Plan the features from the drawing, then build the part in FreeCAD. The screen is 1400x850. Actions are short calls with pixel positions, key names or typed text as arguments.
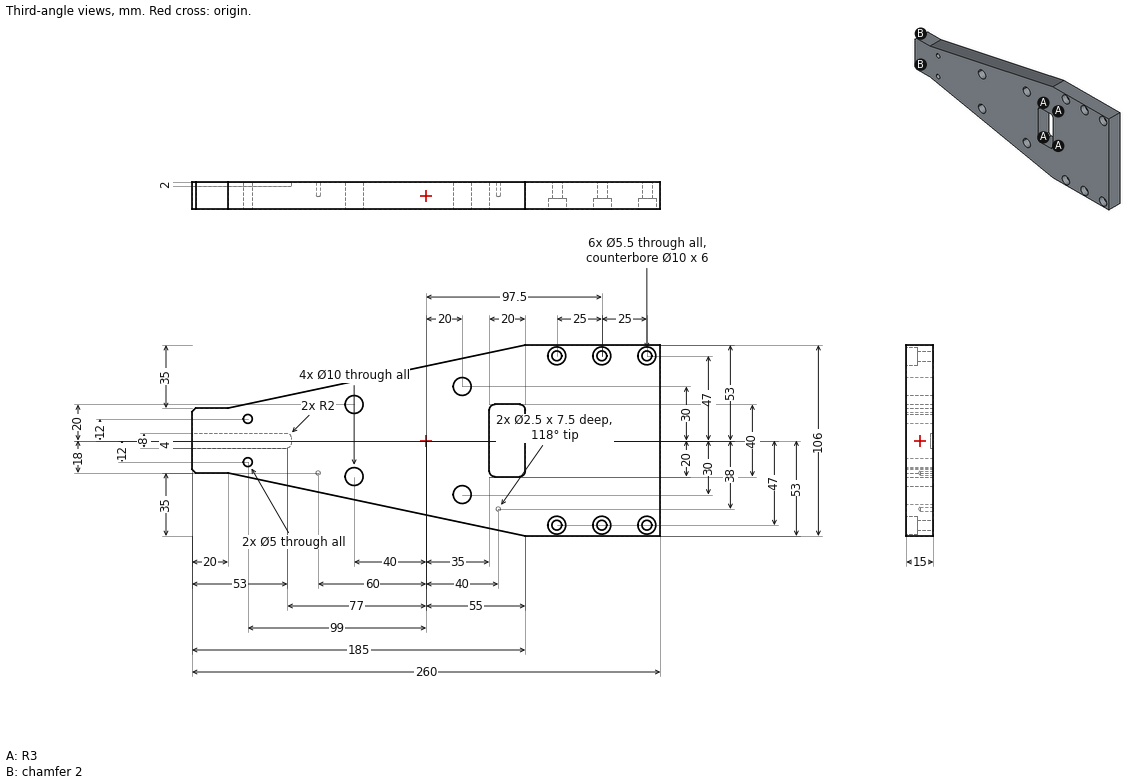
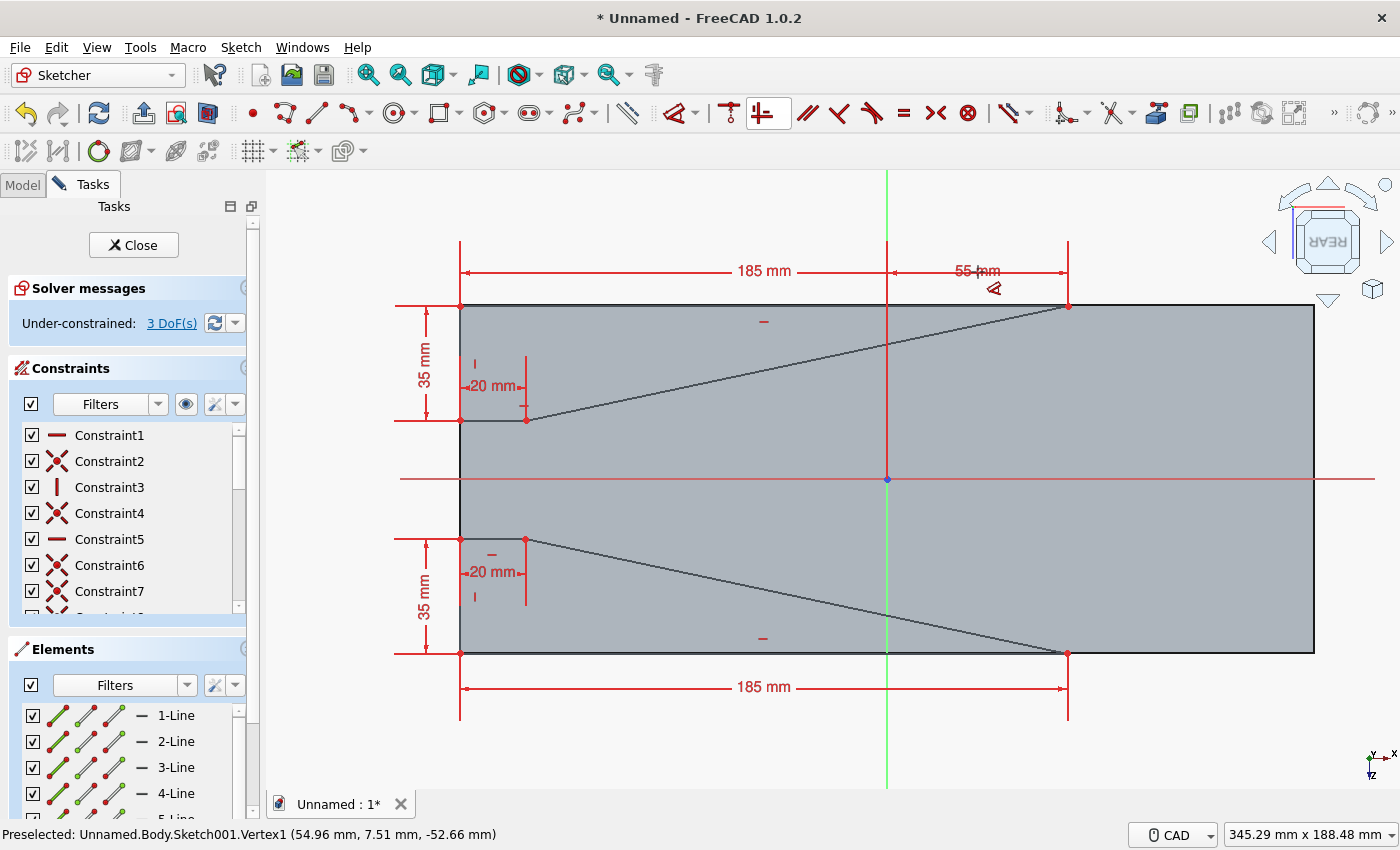
click(1068, 306)
click(1102, 393)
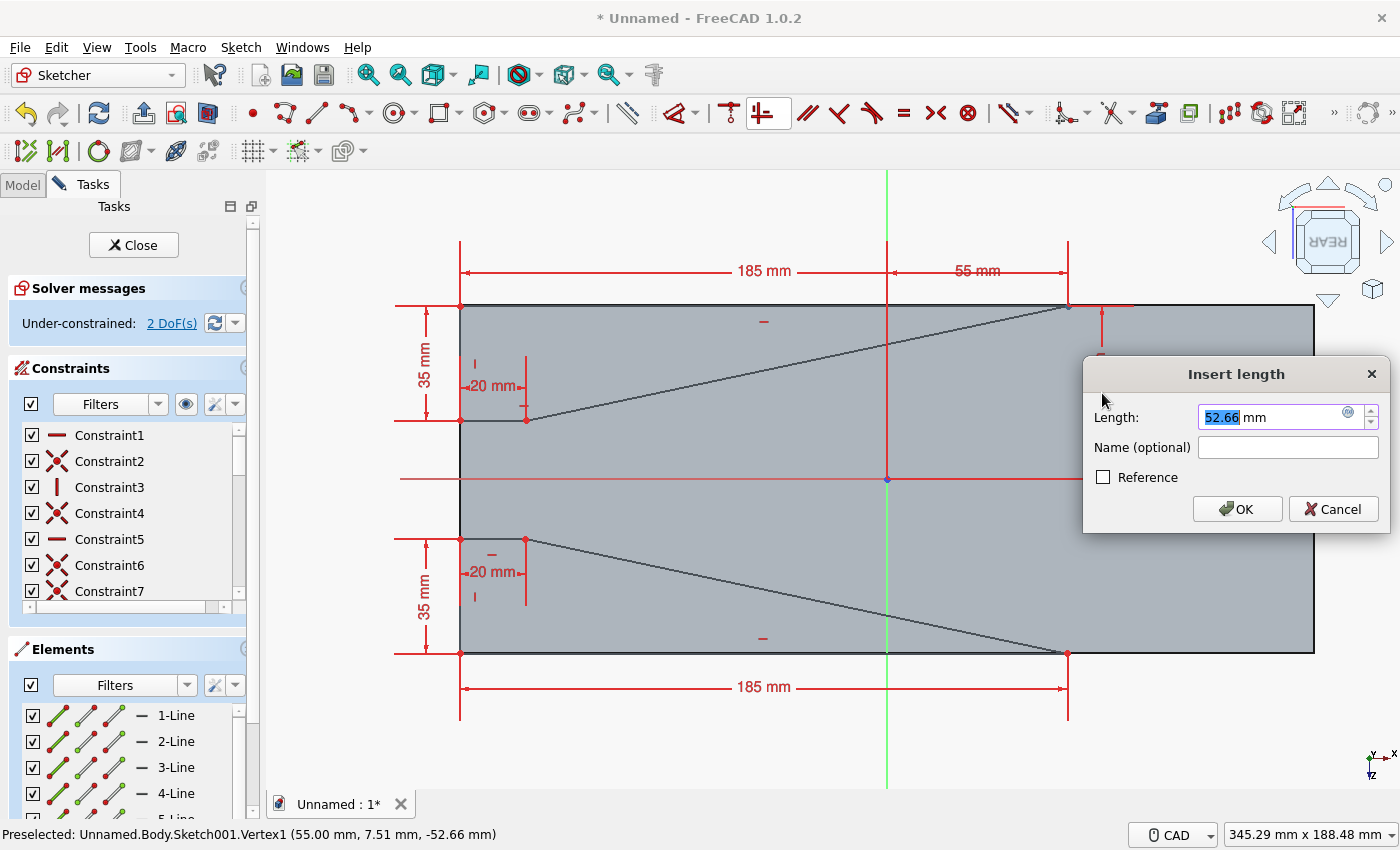
text(53)
key(Return)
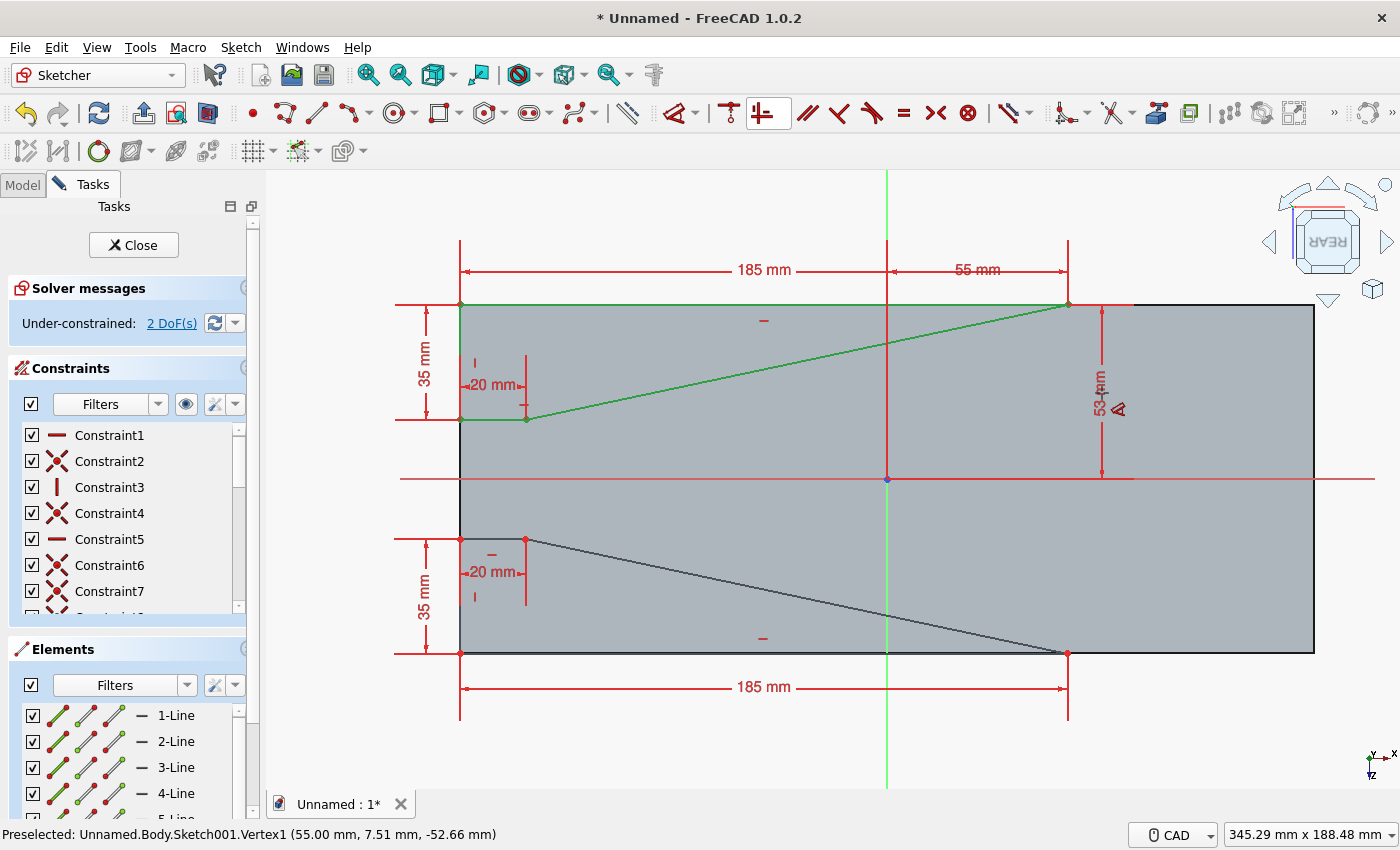
click(1068, 654)
click(978, 688)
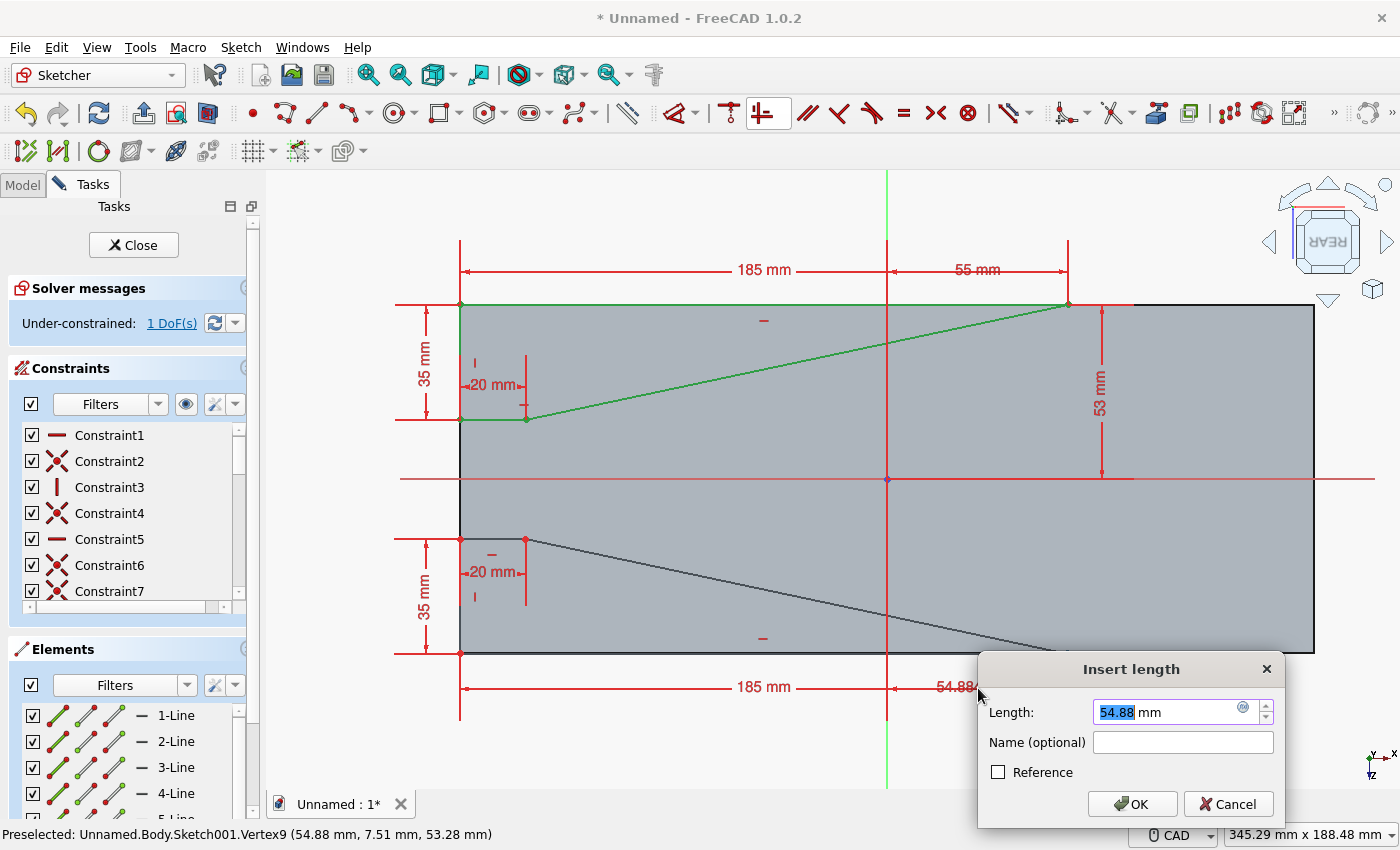
text(55)
key(Return)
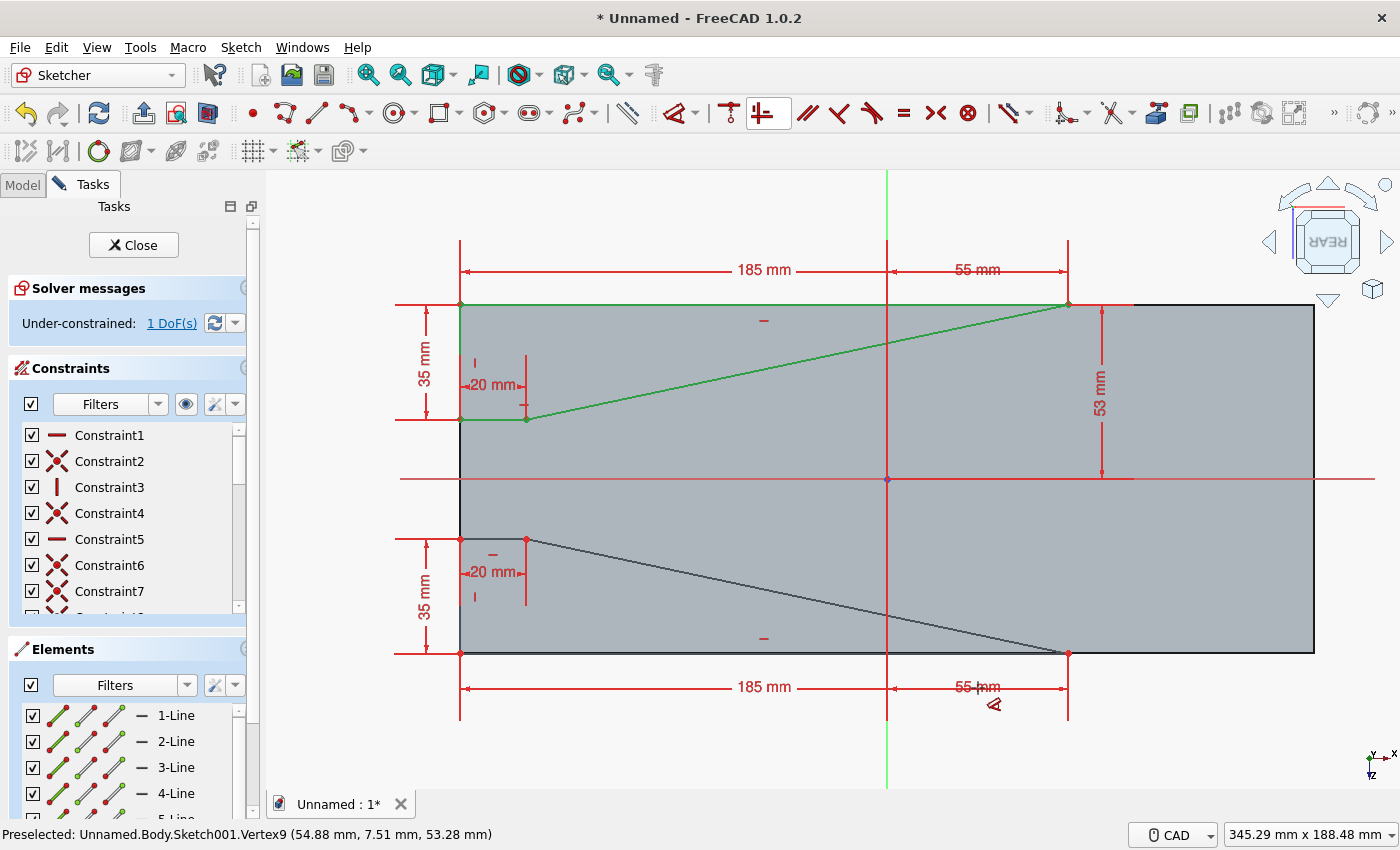
click(1068, 654)
click(1102, 567)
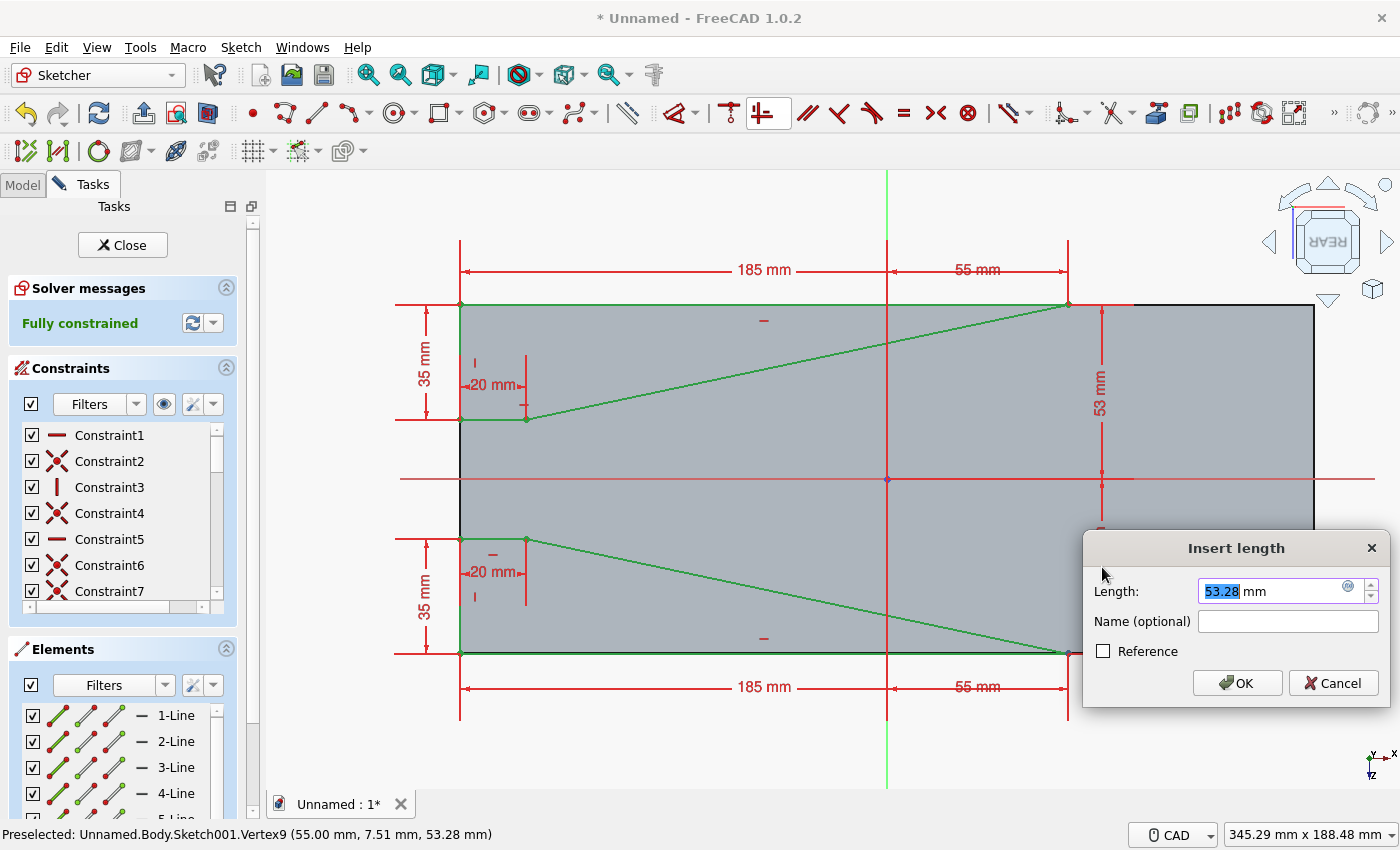
text(53)
key(Return)
key(Escape)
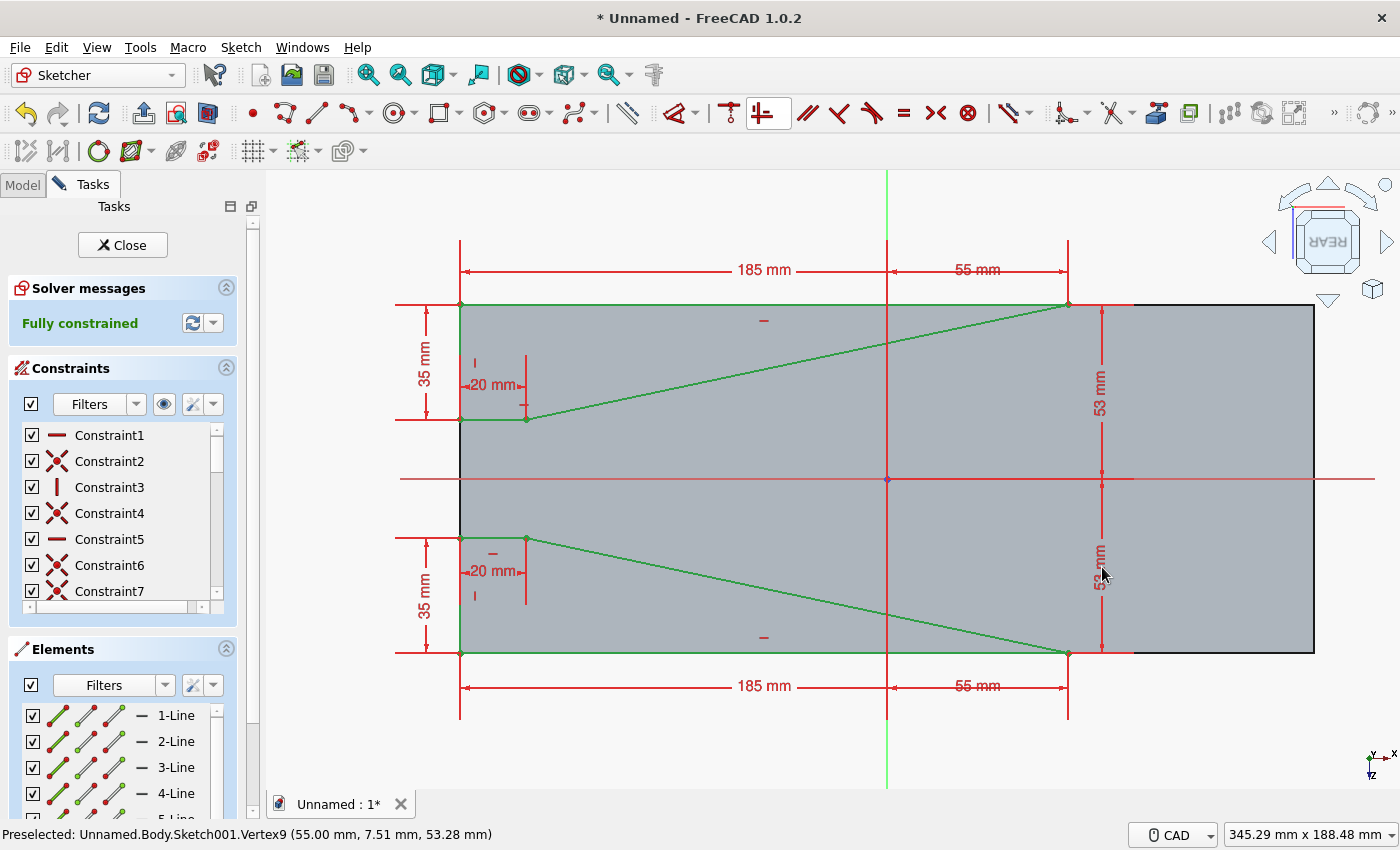
click(123, 245)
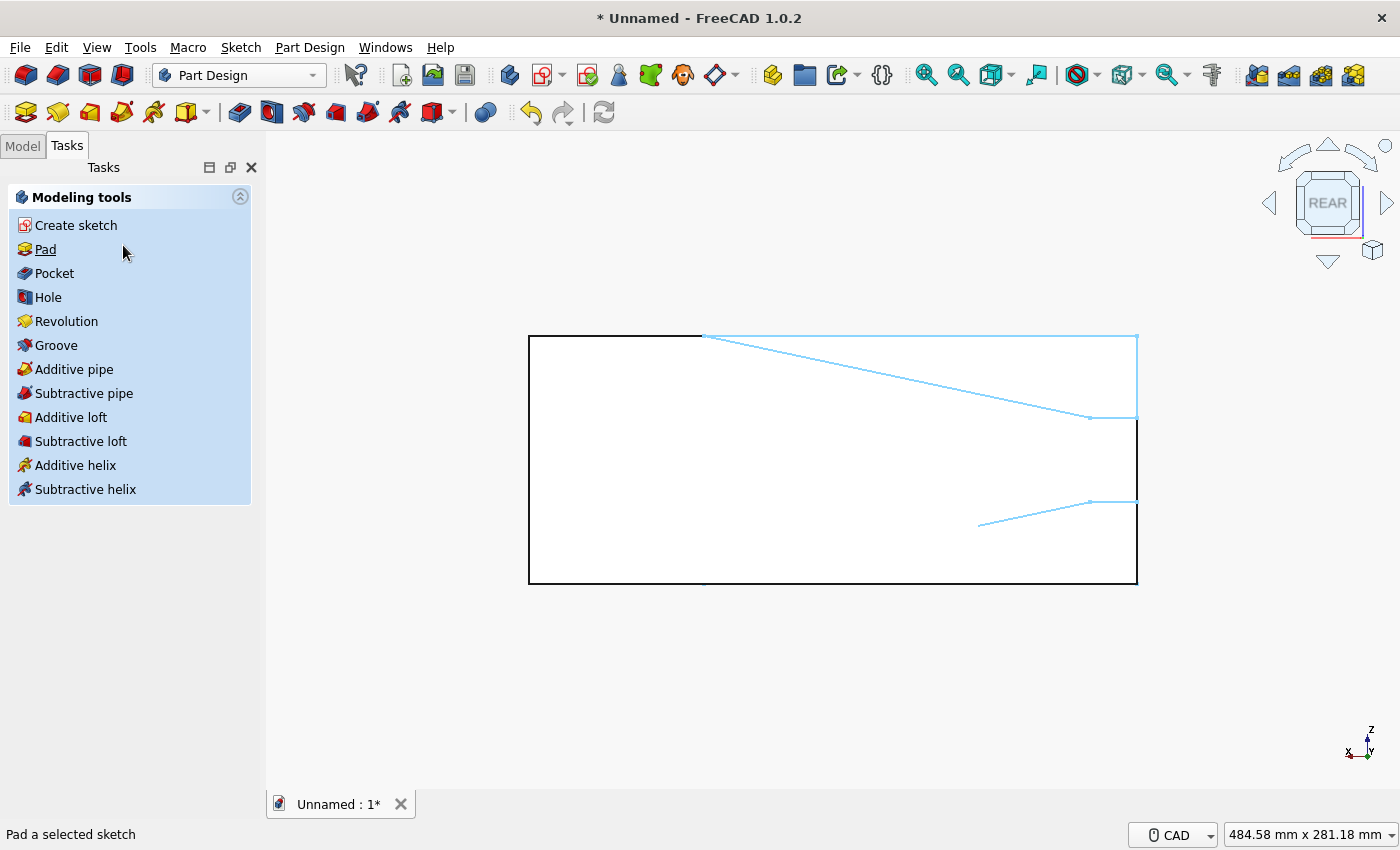
click(240, 112)